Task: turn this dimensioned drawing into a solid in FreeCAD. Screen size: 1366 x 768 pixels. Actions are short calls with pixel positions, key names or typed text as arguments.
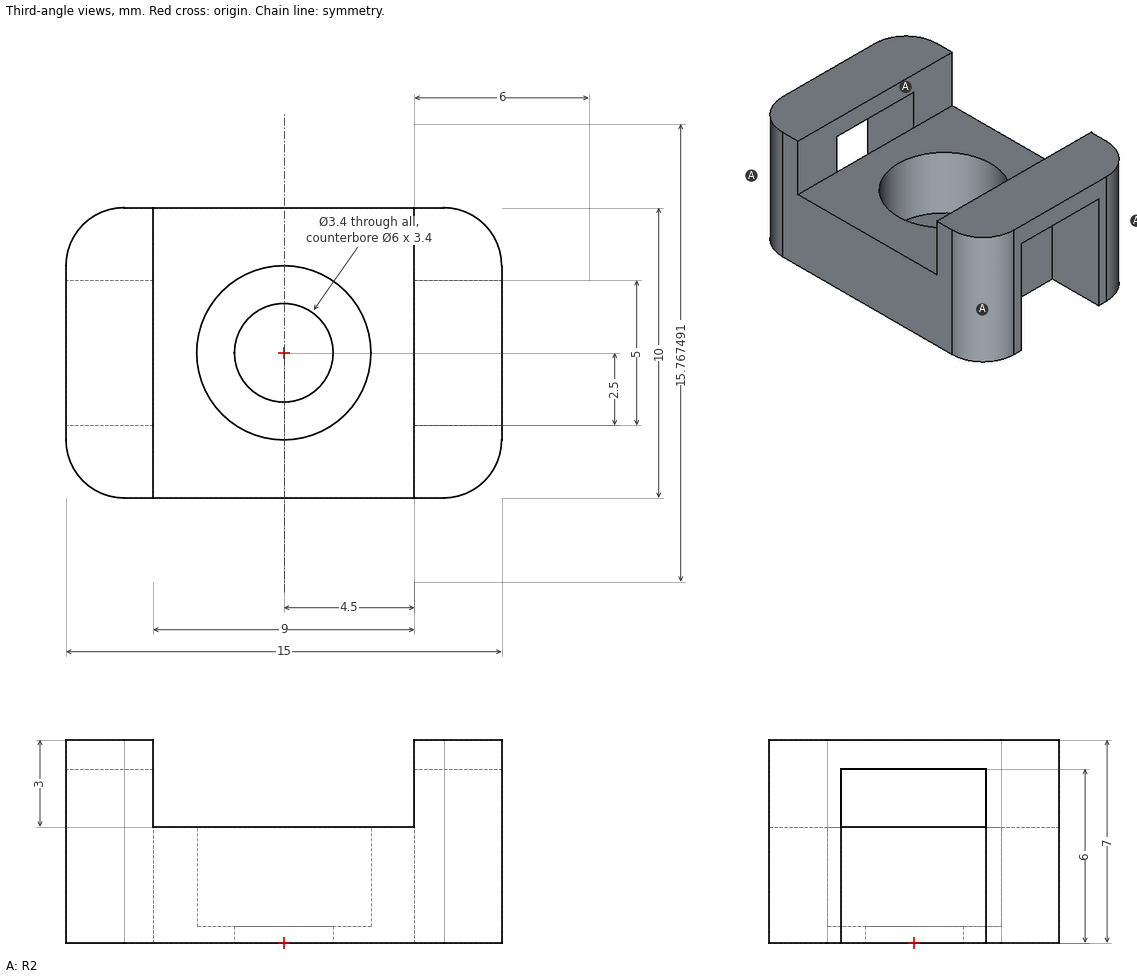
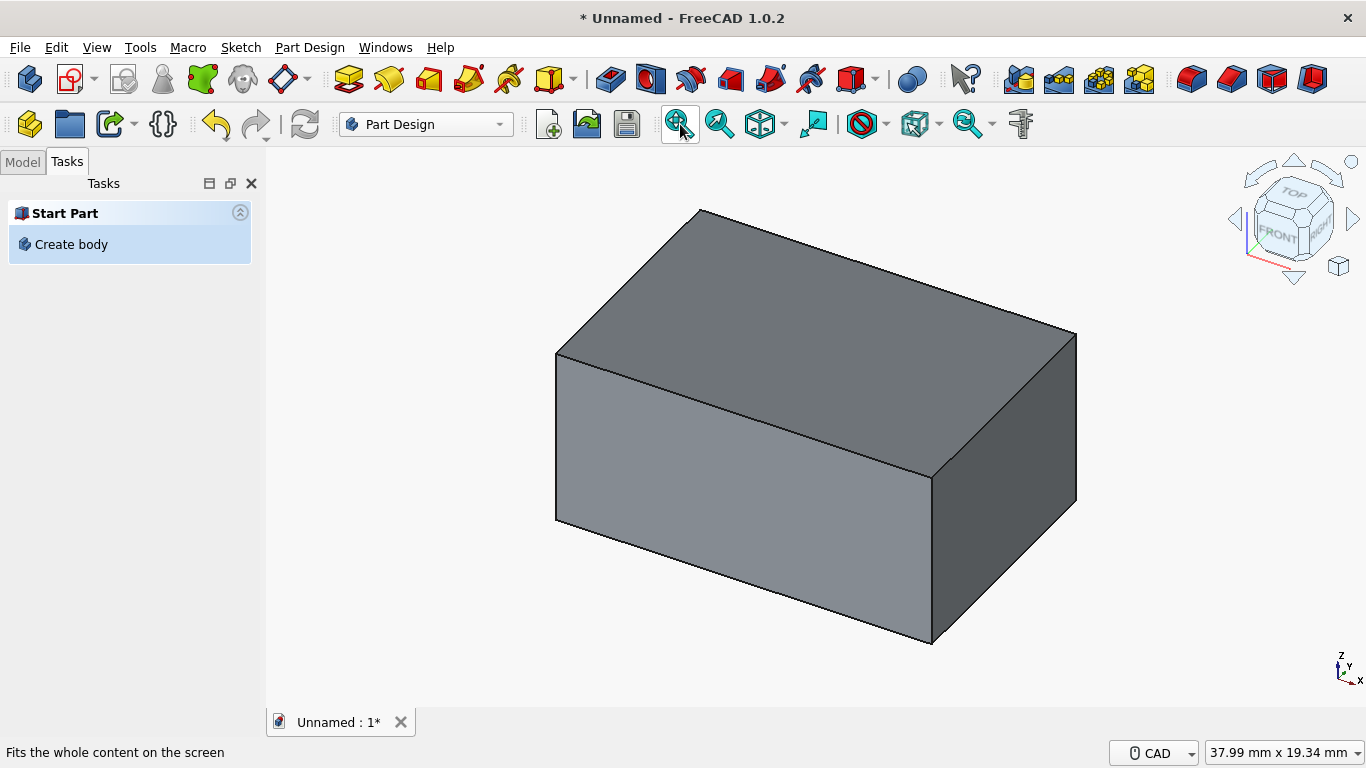
click(870, 361)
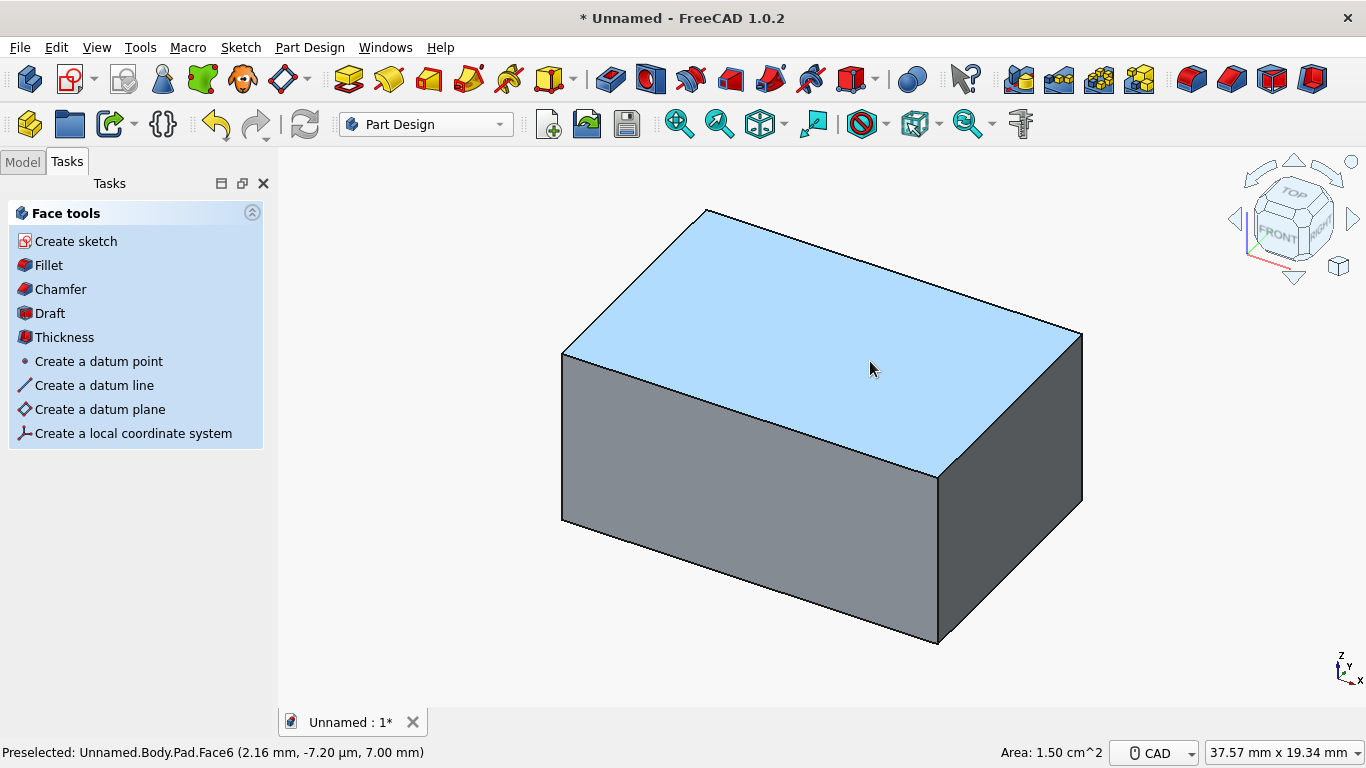
click(70, 80)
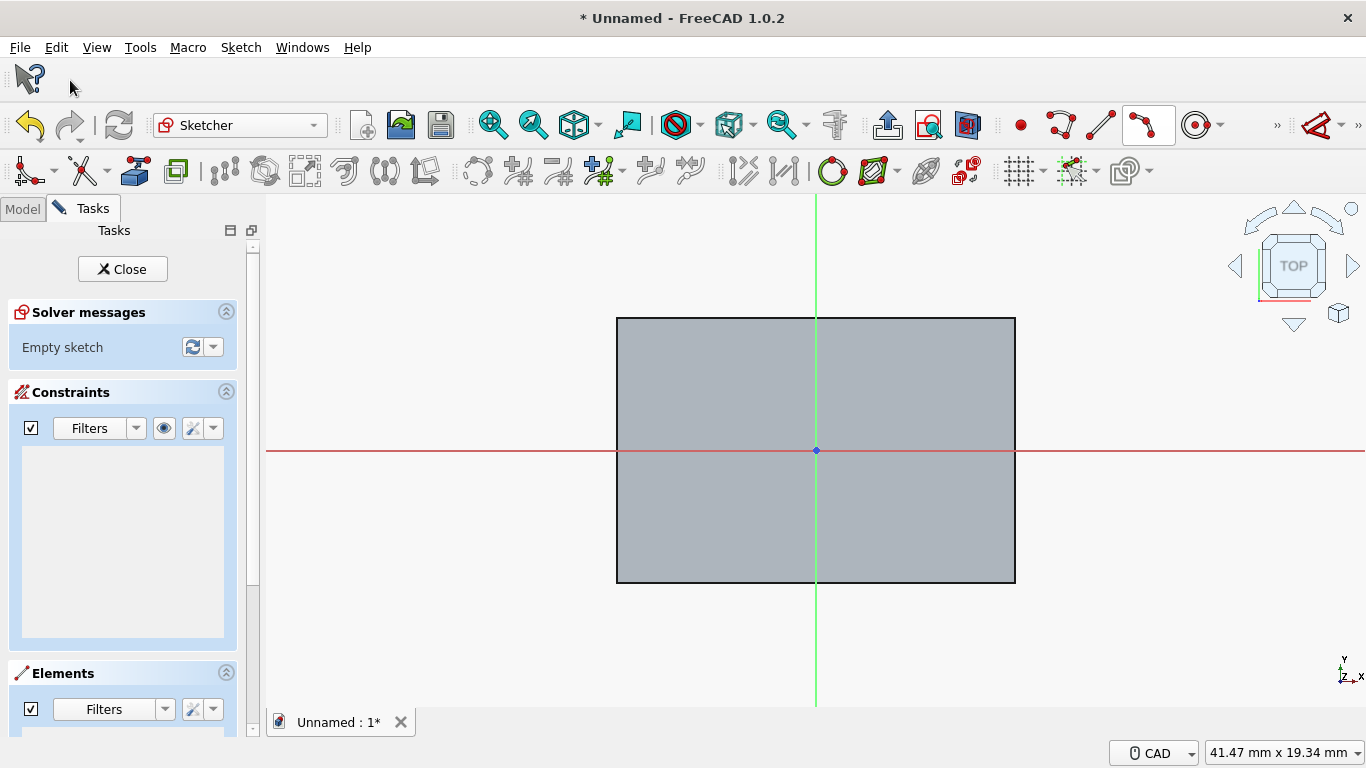
scroll(438, 450, down, 1)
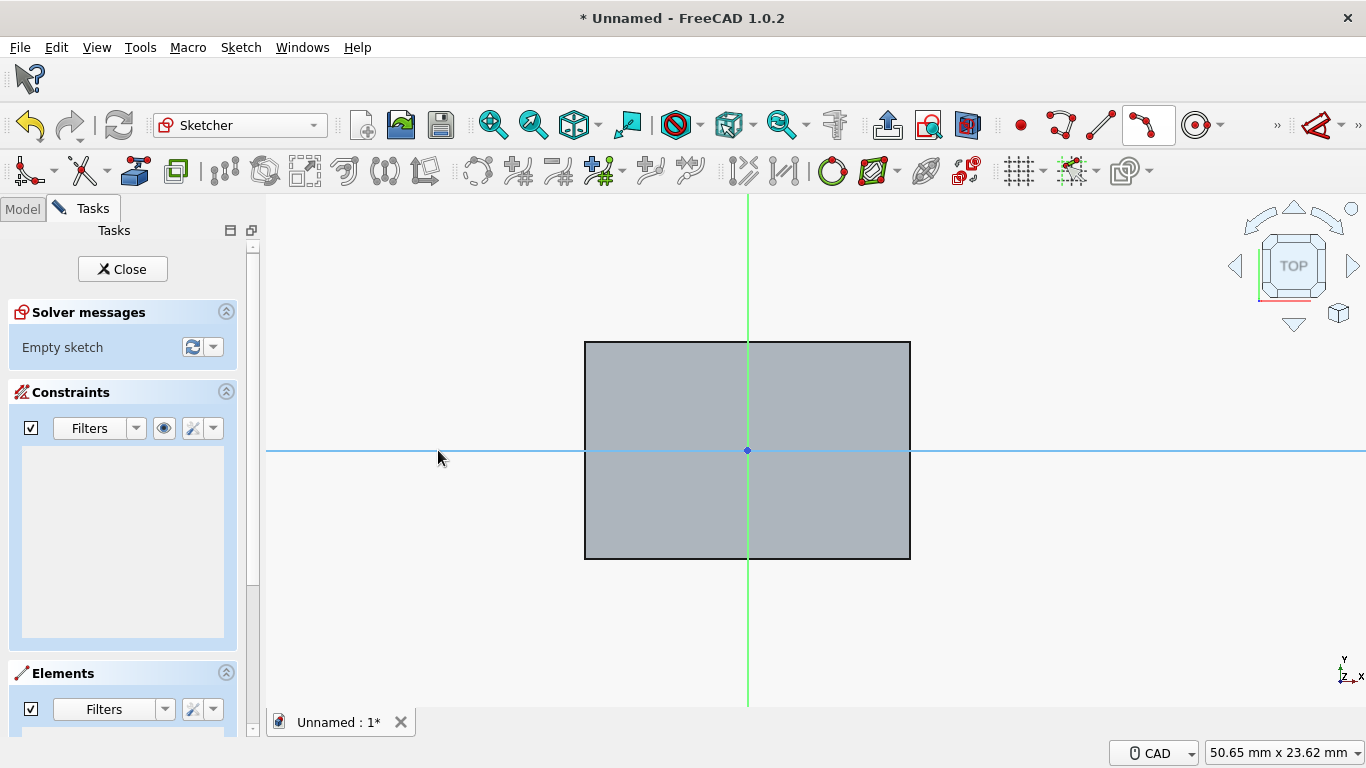
key(g)
key(v)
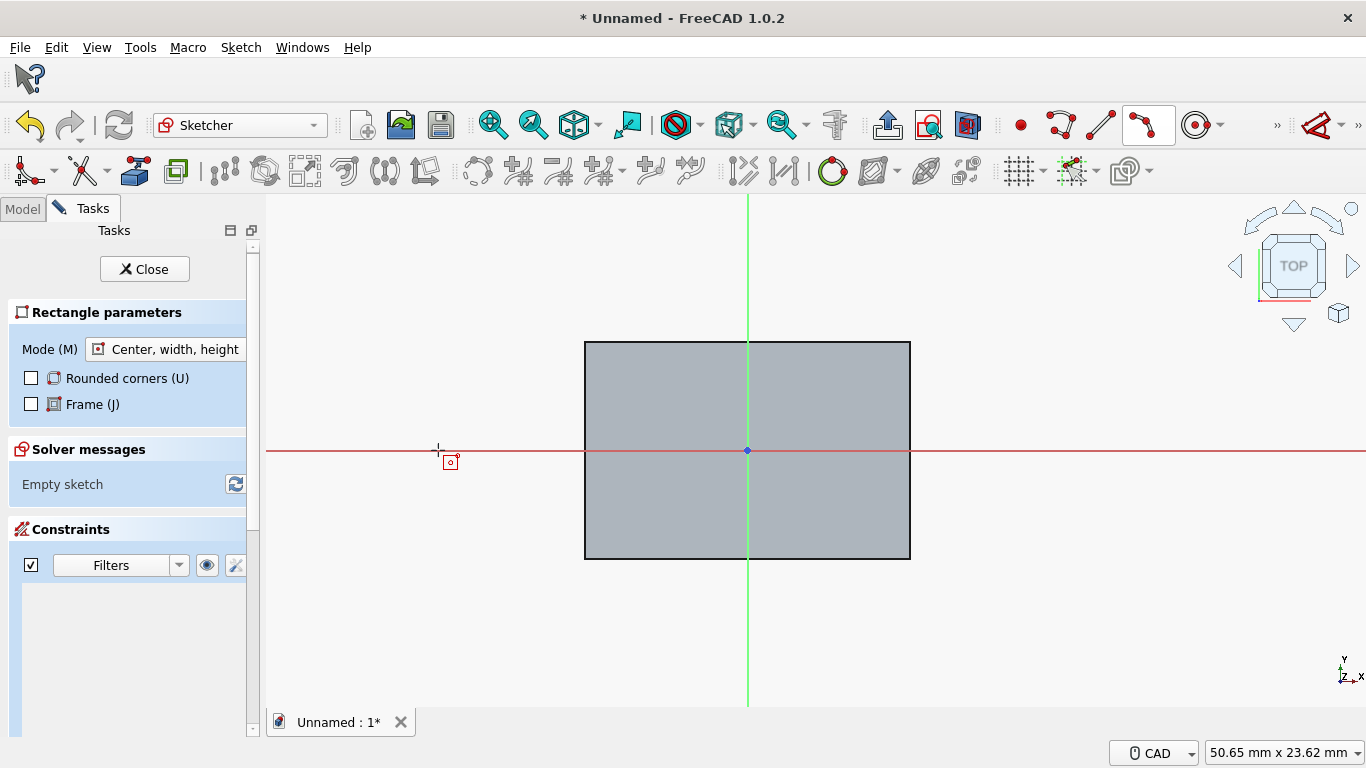
click(748, 450)
click(845, 279)
key(Escape)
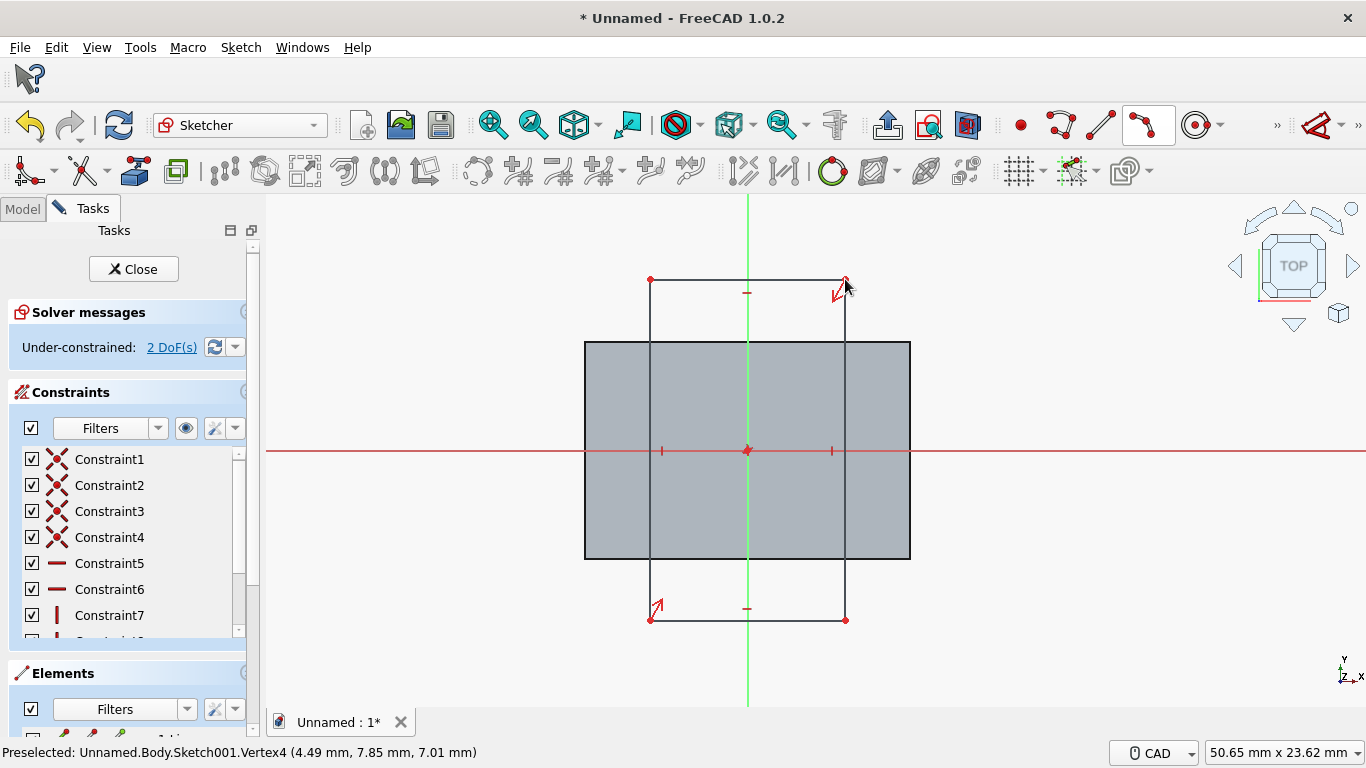
click(709, 621)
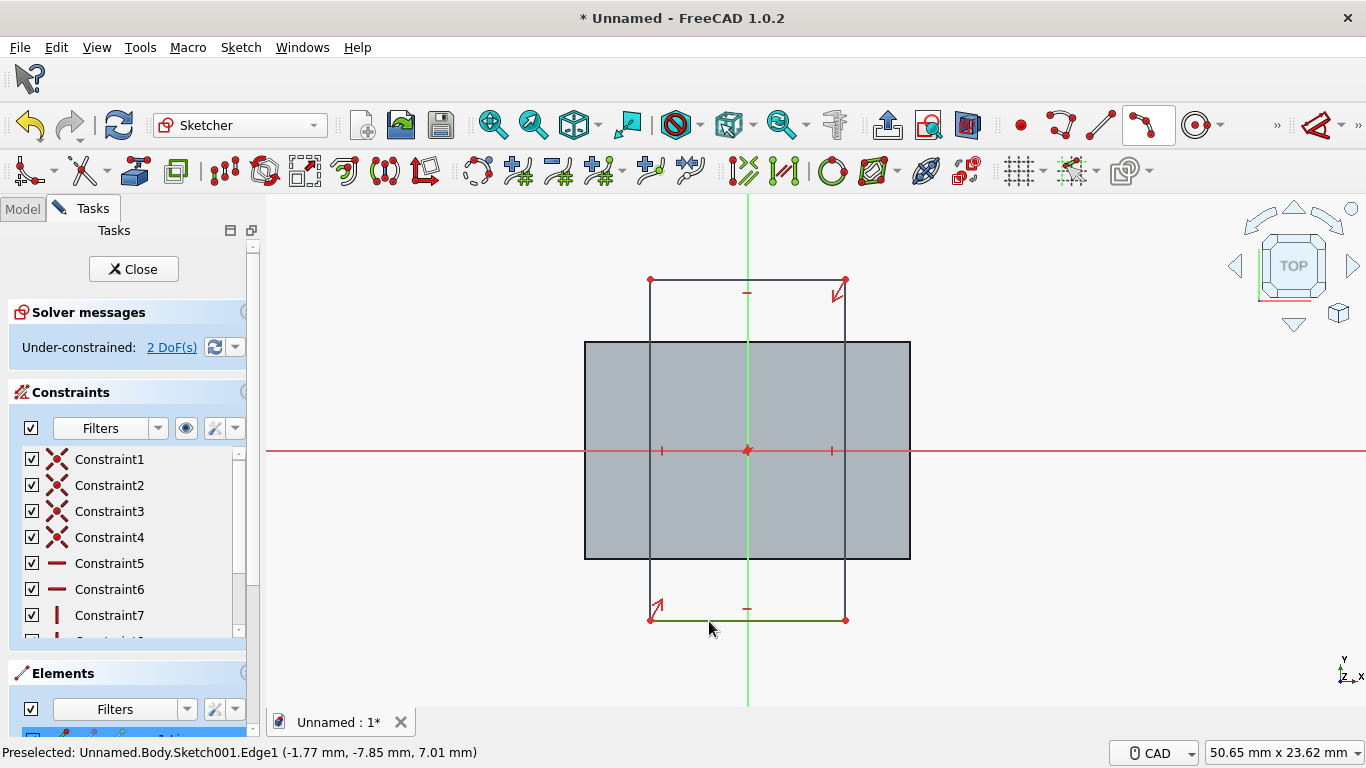
key(l)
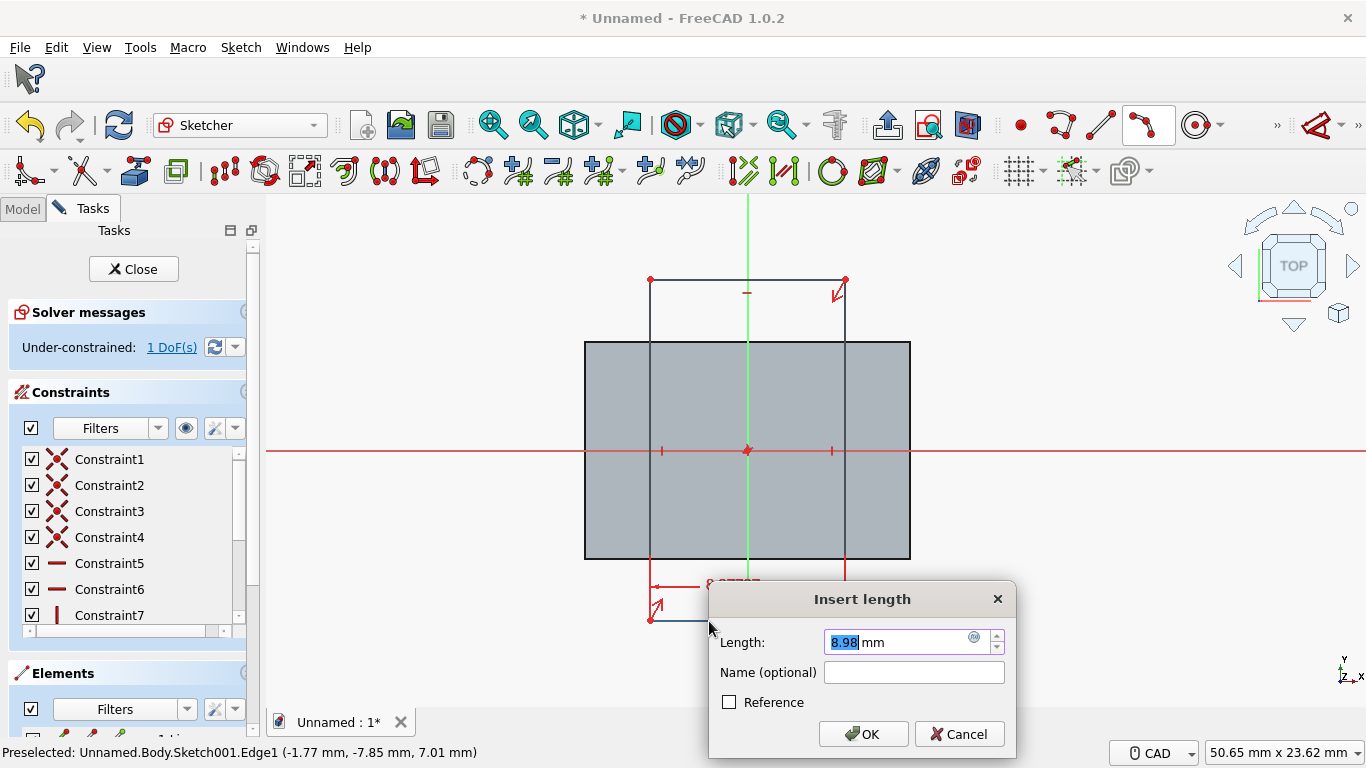
text(9)
key(Return)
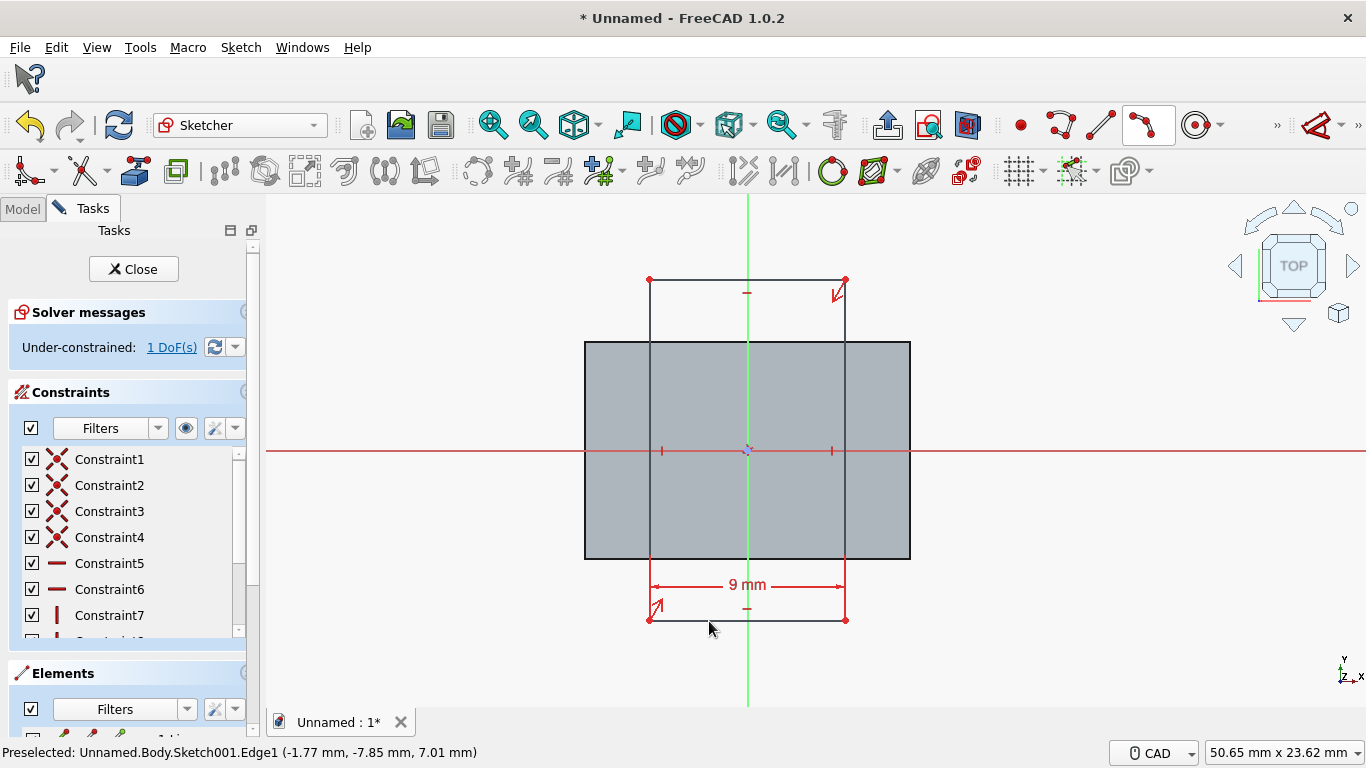
click(845, 519)